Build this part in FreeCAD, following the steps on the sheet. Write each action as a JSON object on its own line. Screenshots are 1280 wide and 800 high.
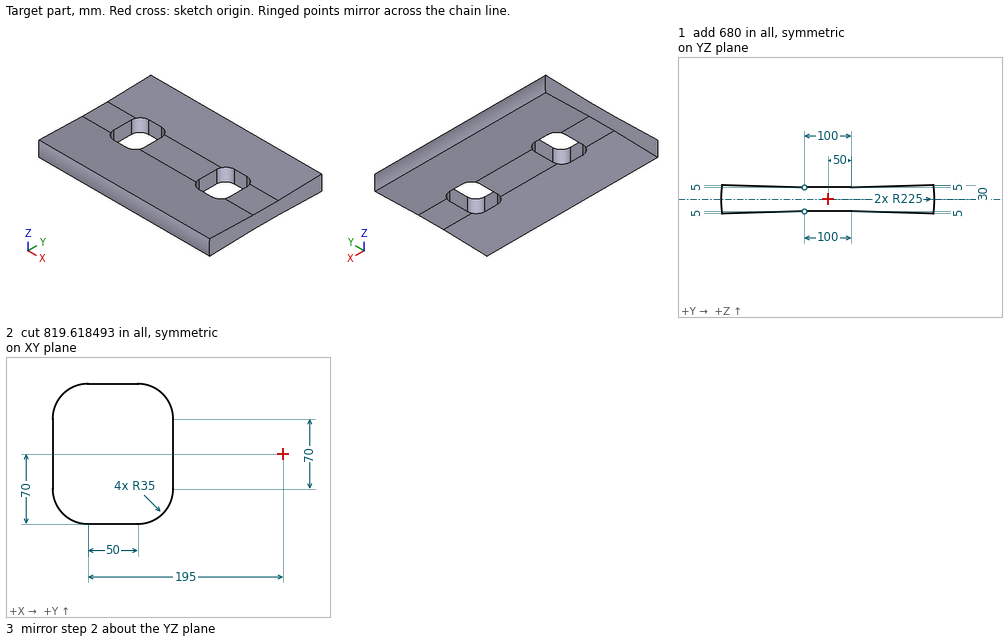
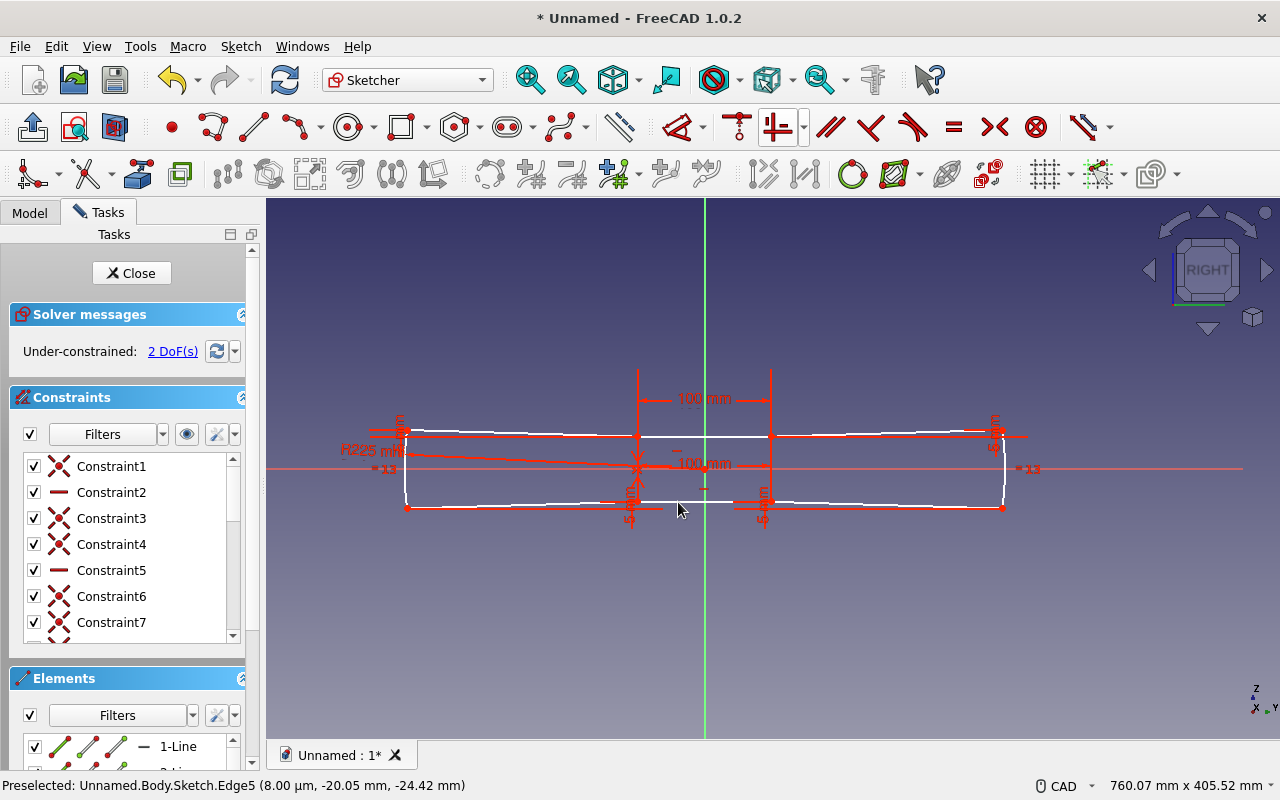
{"action": "left_click", "coordinate": [1002, 430]}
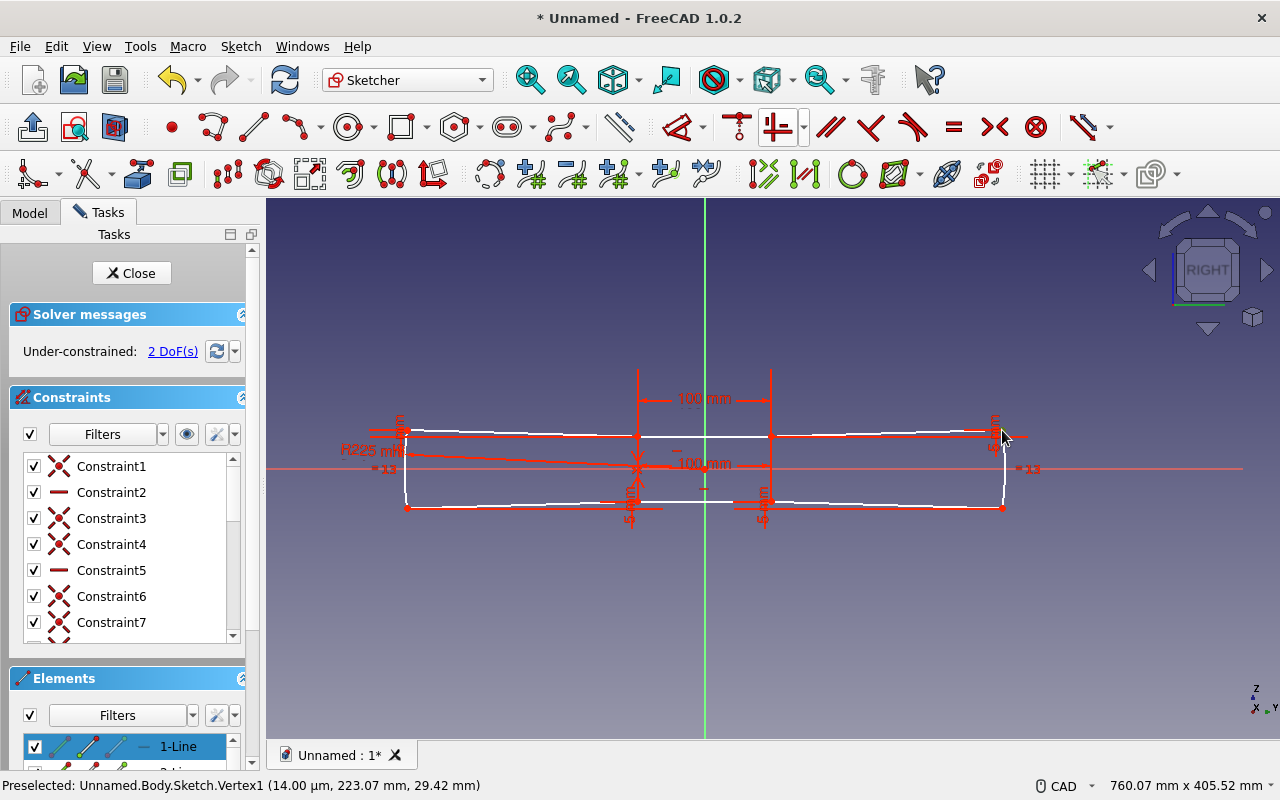
{"action": "key", "text": "i"}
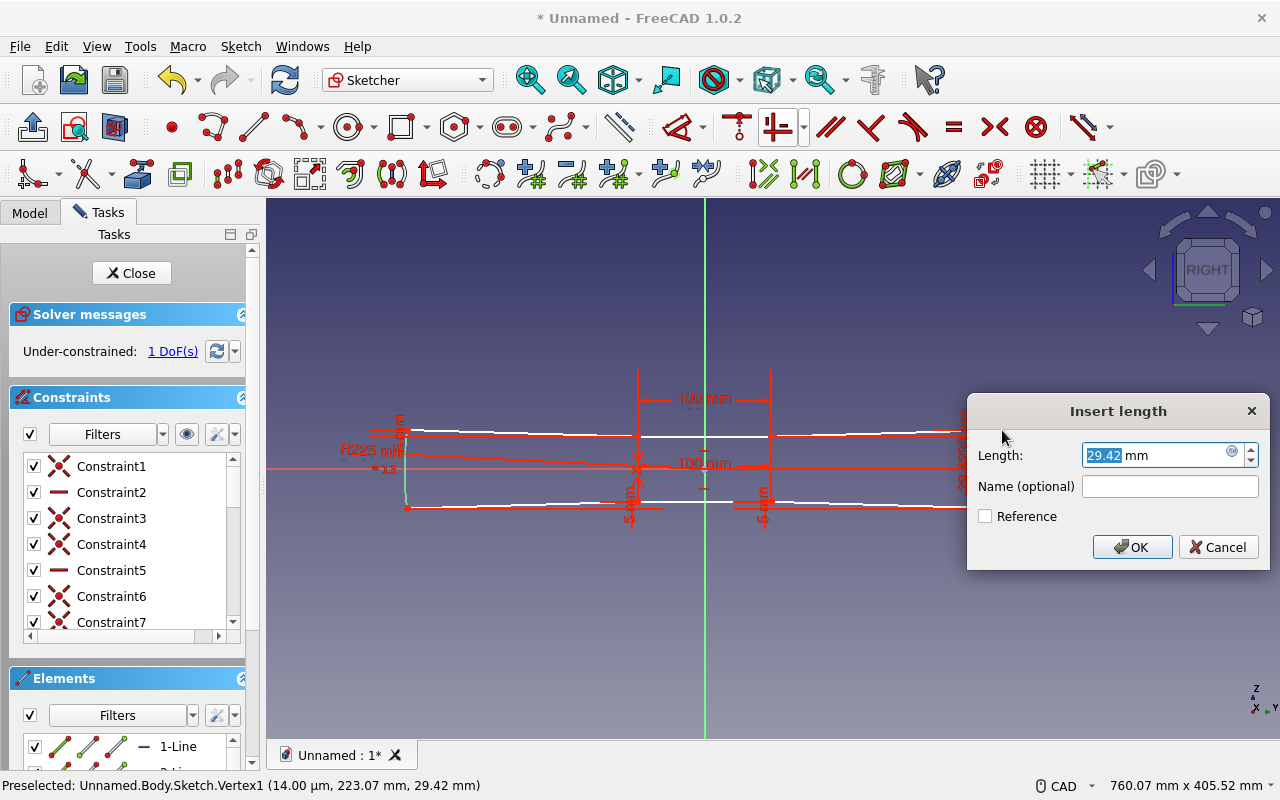
{"action": "type", "text": "30"}
{"action": "key", "text": "Return"}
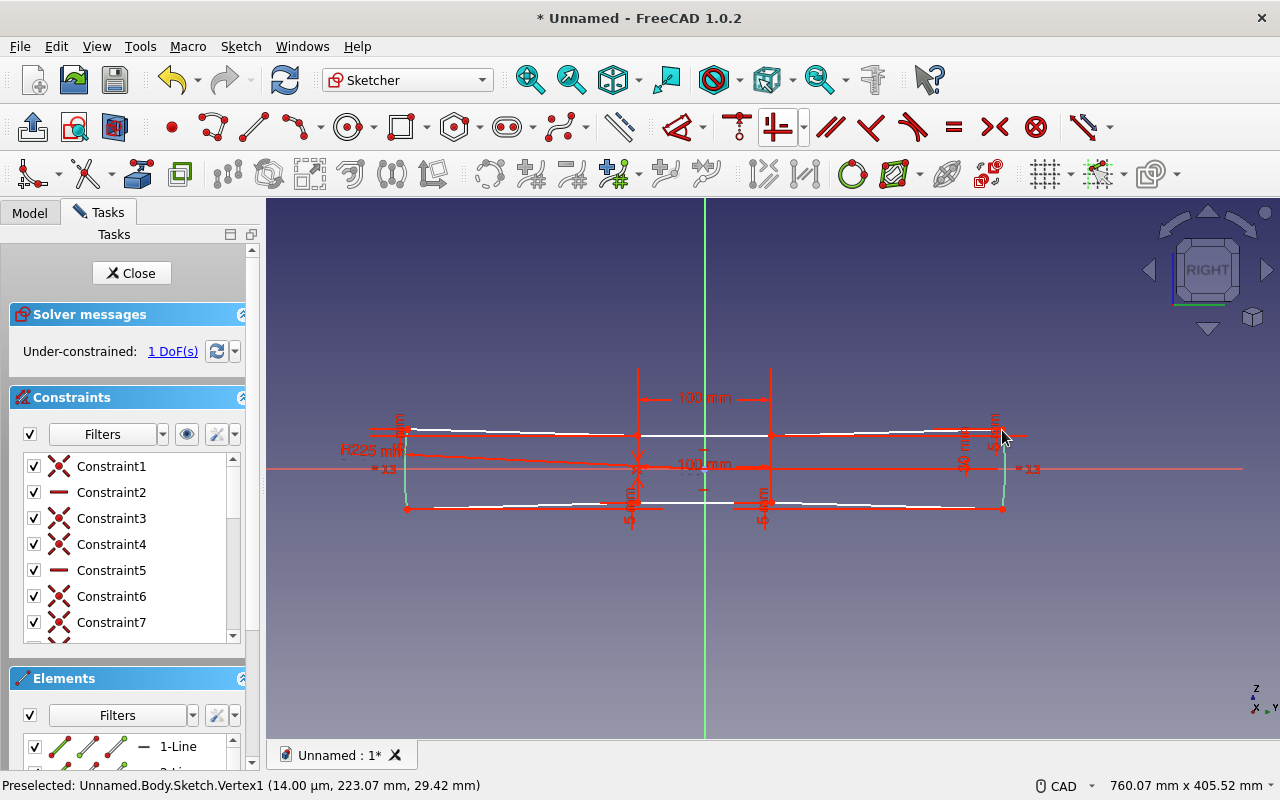
{"action": "left_click", "coordinate": [771, 436]}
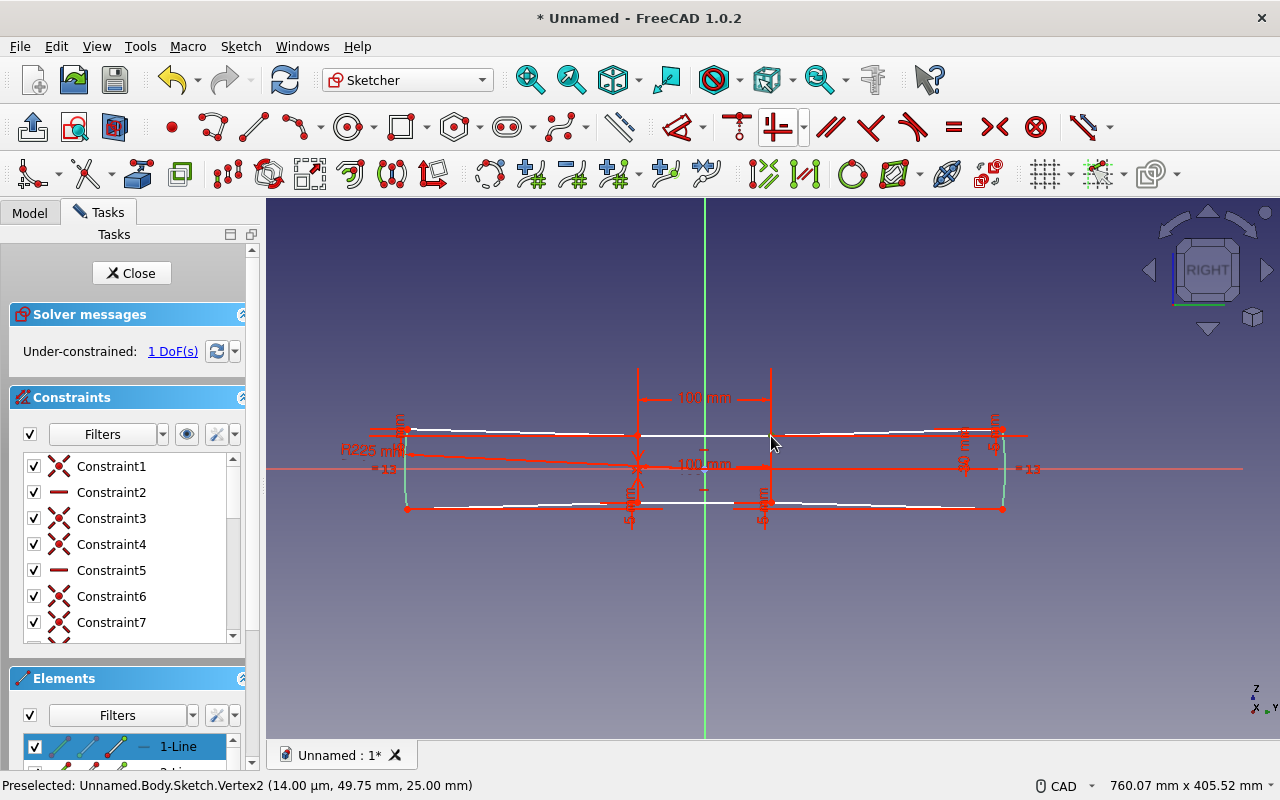
{"action": "key", "text": "l"}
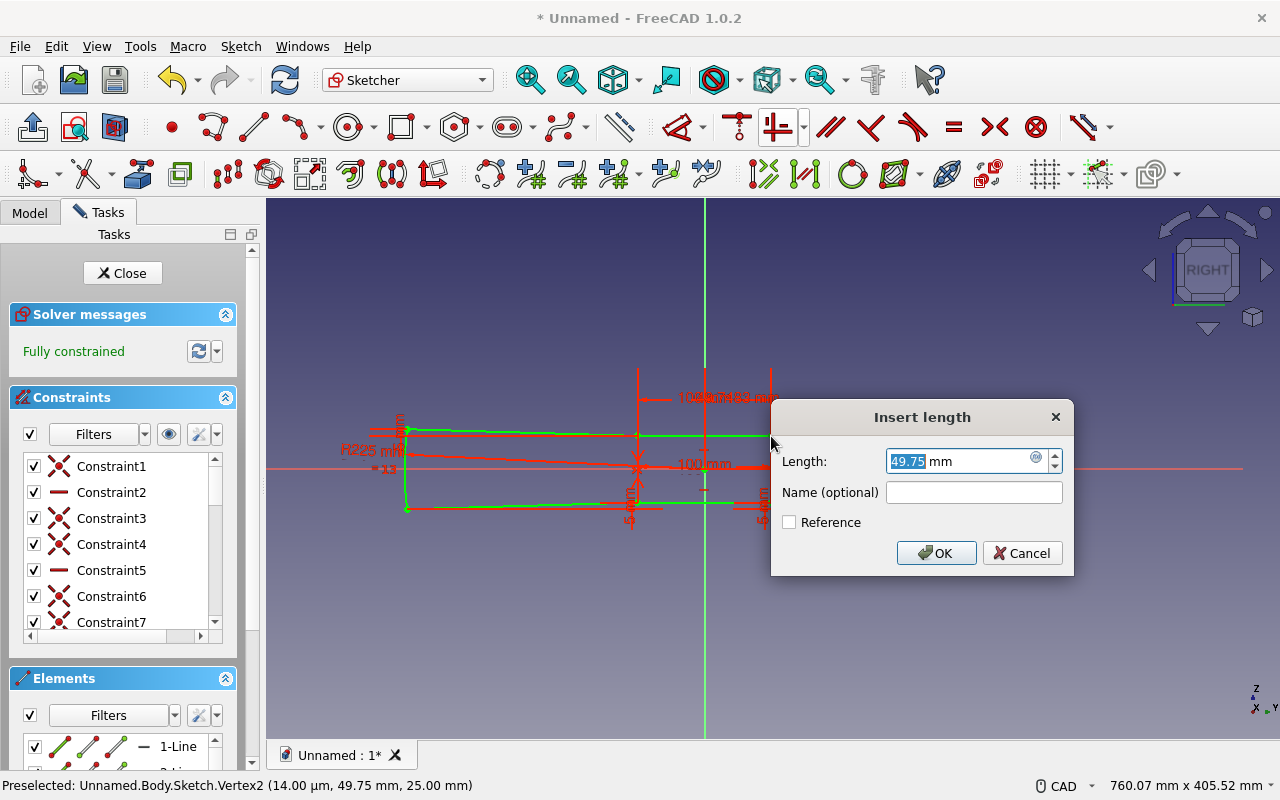
{"action": "type", "text": "50"}
{"action": "key", "text": "Return"}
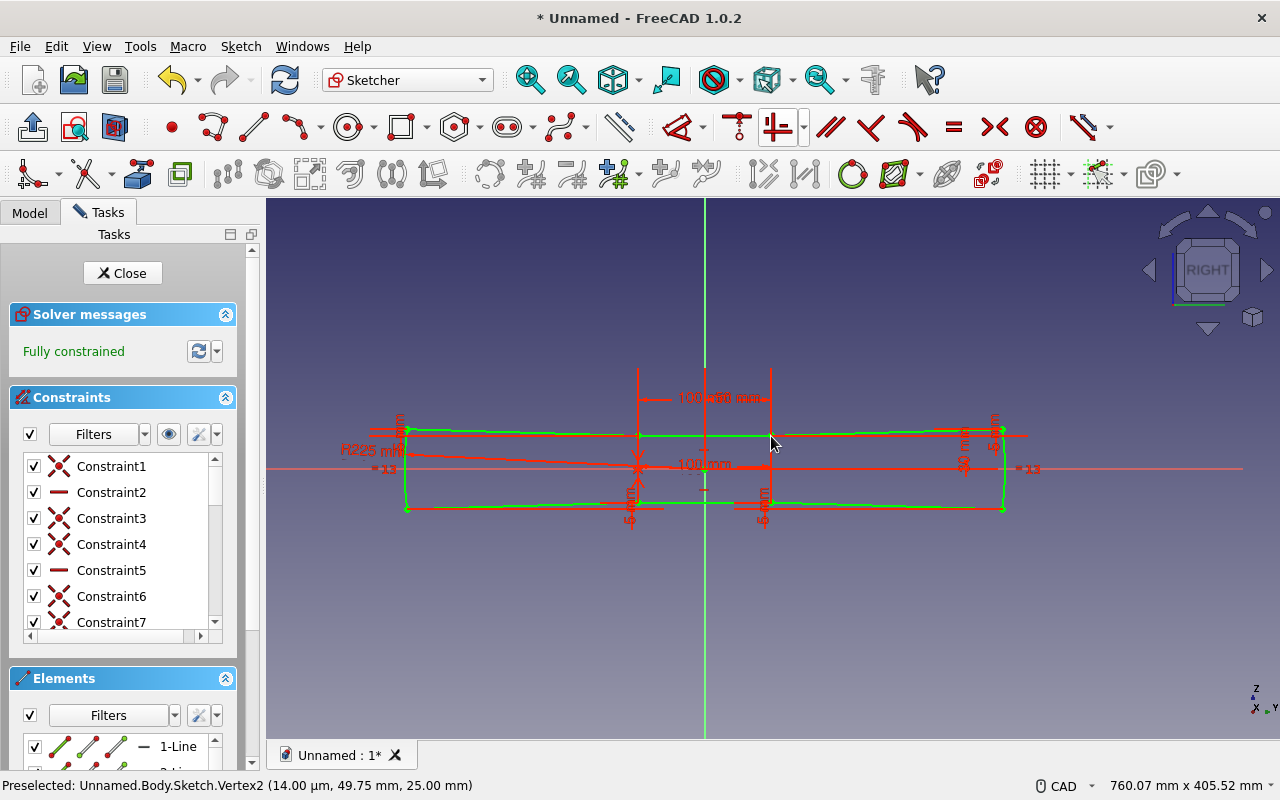
{"action": "left_click", "coordinate": [123, 273]}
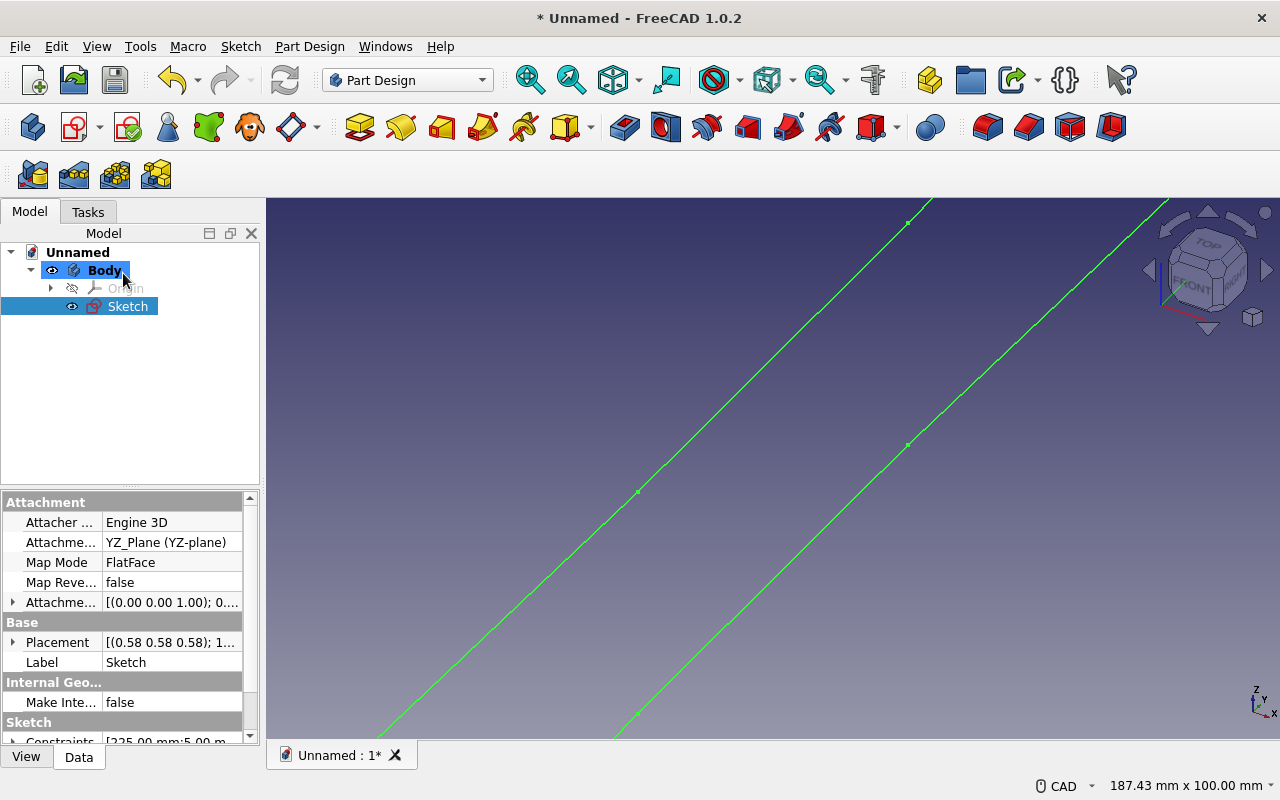
{"action": "left_click", "coordinate": [360, 128]}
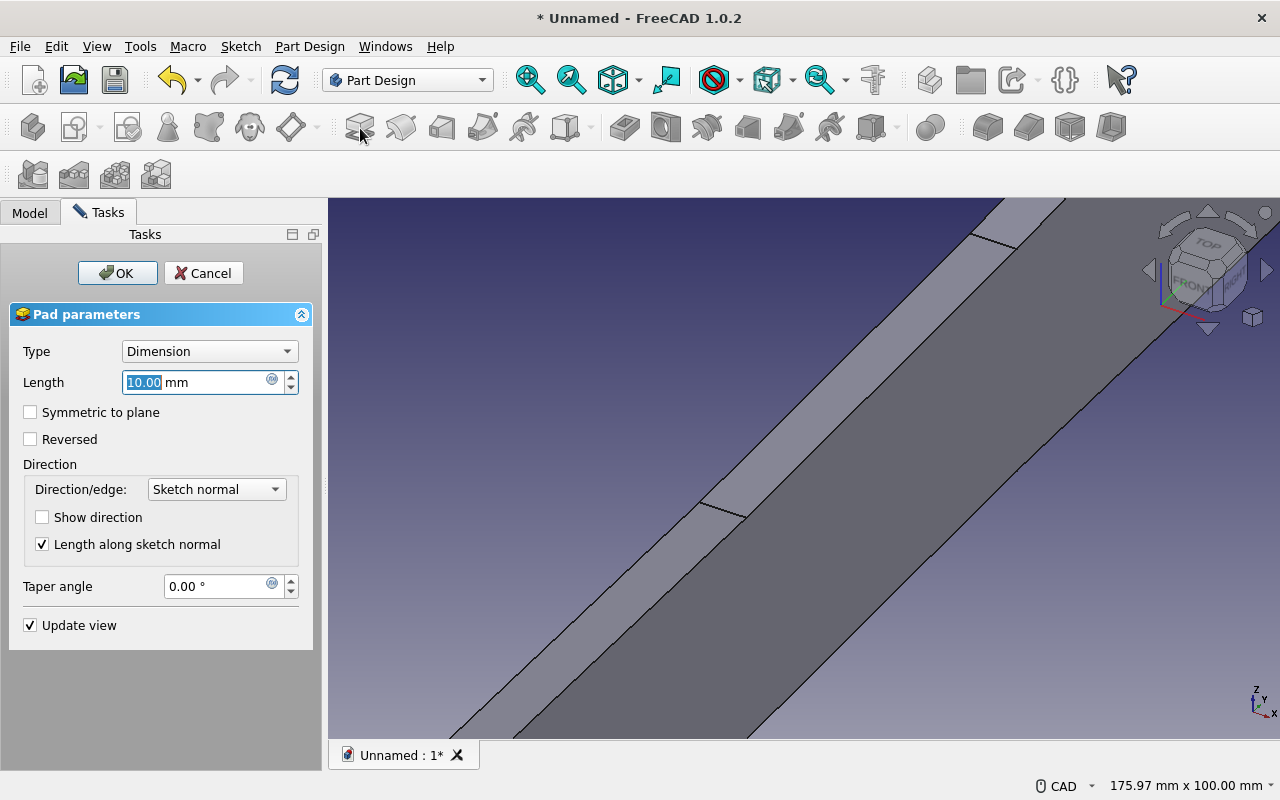
{"action": "type", "text": "680"}
{"action": "key", "text": "Tab"}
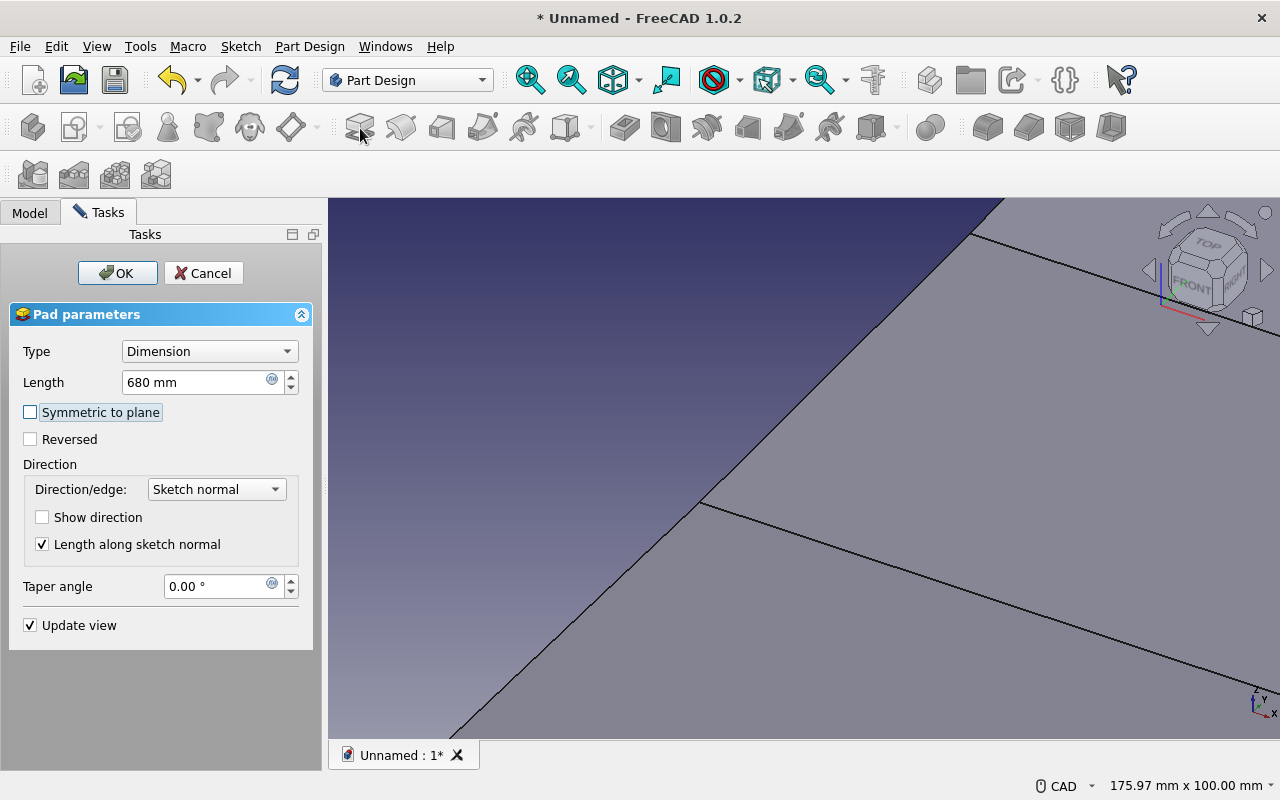
{"action": "left_click", "coordinate": [31, 412]}